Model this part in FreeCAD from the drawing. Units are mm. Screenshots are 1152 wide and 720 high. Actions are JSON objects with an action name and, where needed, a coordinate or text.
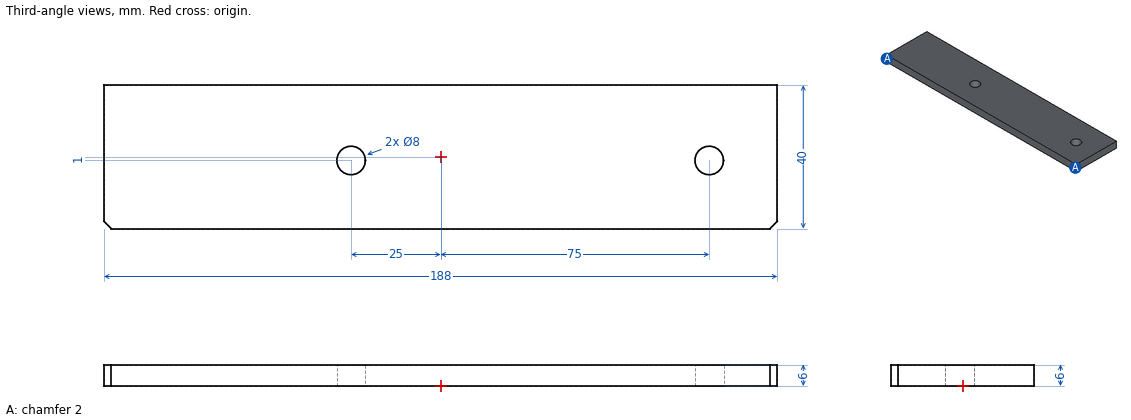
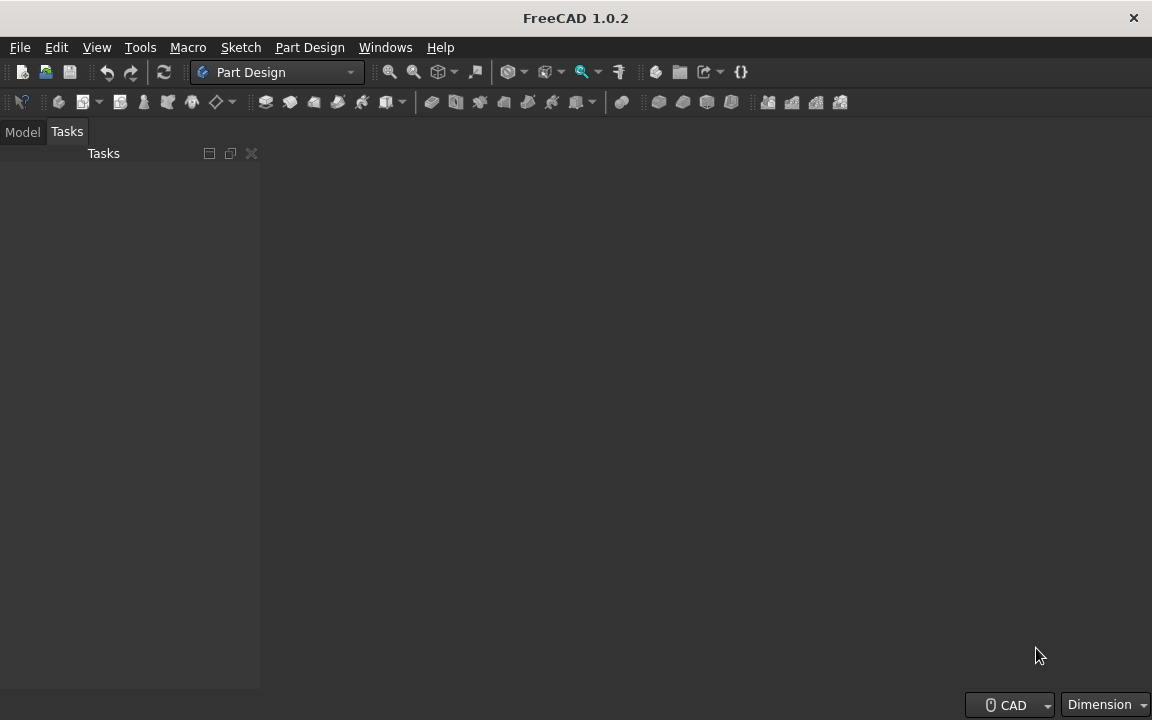
{"action": "key", "text": "ctrl+n"}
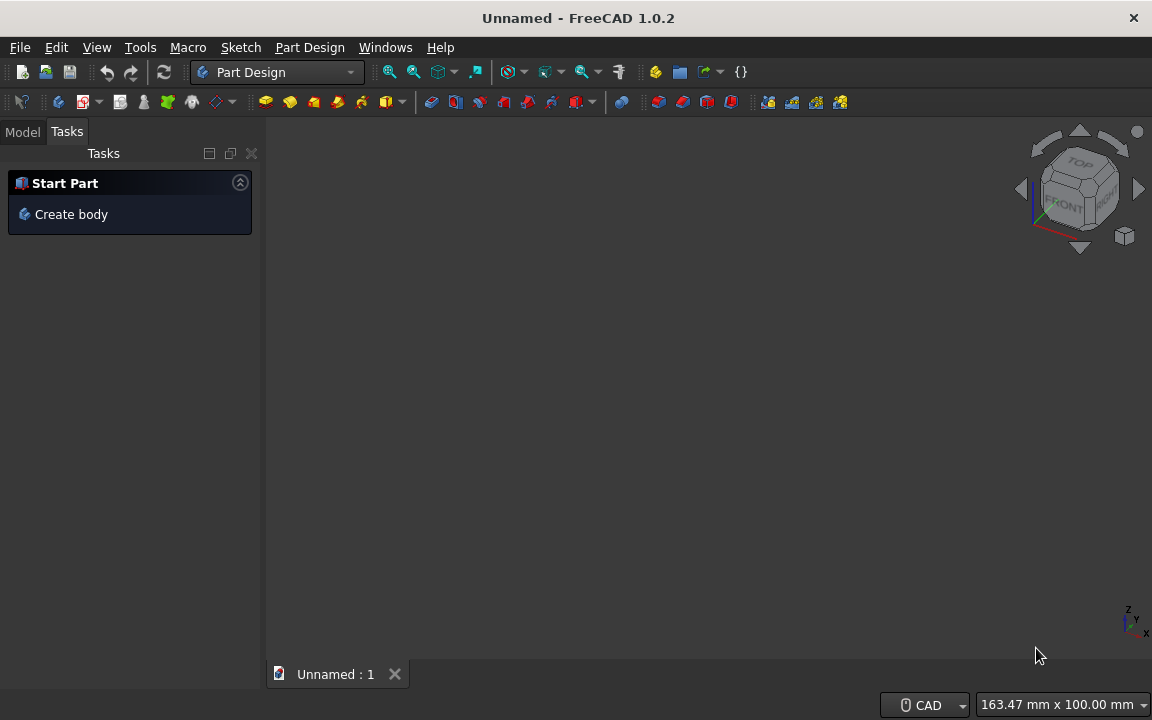
{"action": "left_click", "coordinate": [84, 102]}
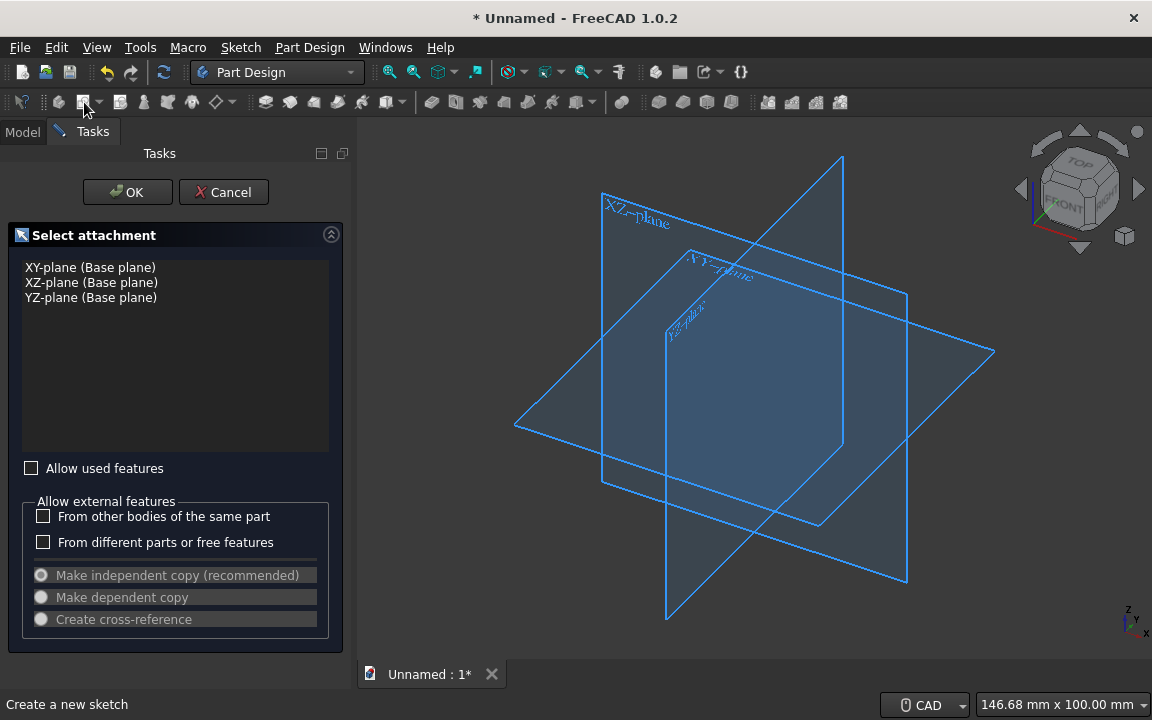
{"action": "left_click", "coordinate": [82, 268]}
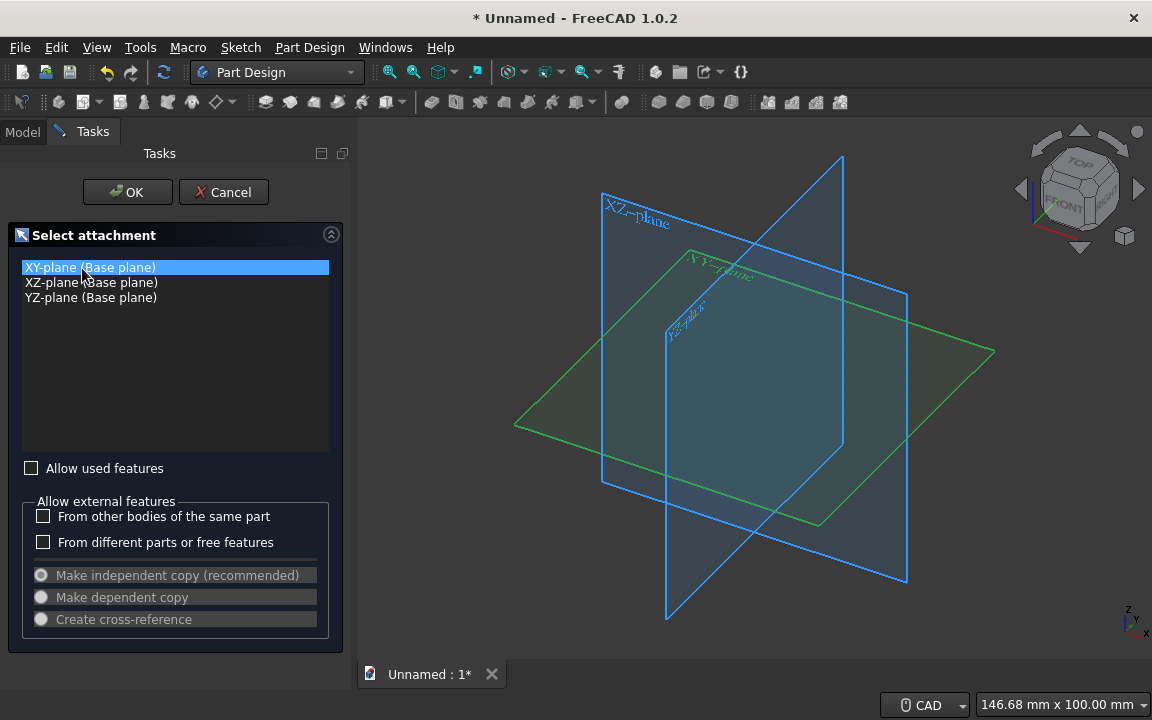
{"action": "left_click", "coordinate": [128, 192]}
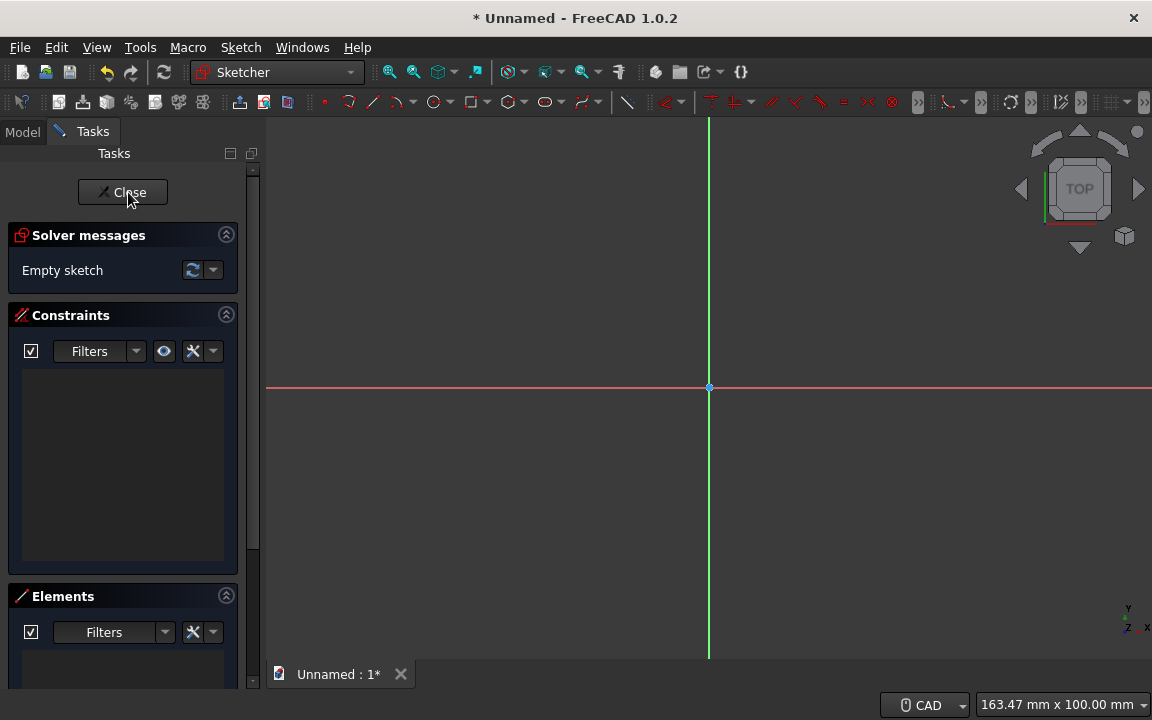
{"action": "scroll", "coordinate": [585, 388], "scroll_direction": "down", "scroll_amount": 4}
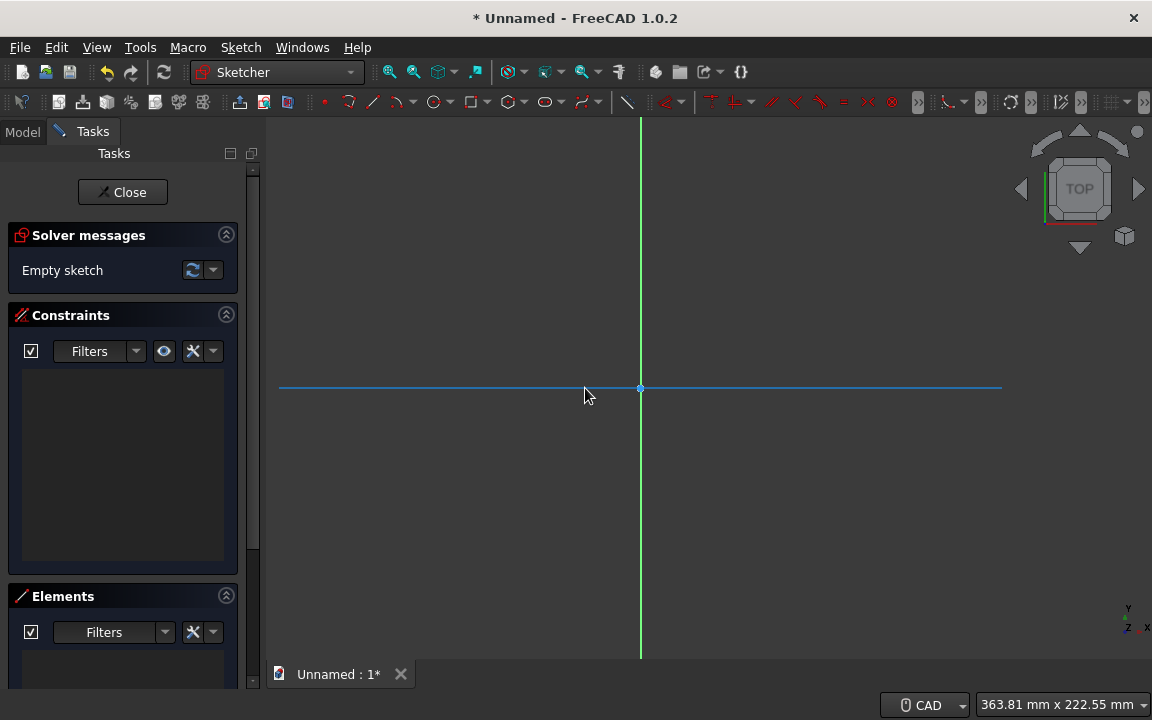
{"action": "left_click", "coordinate": [490, 102]}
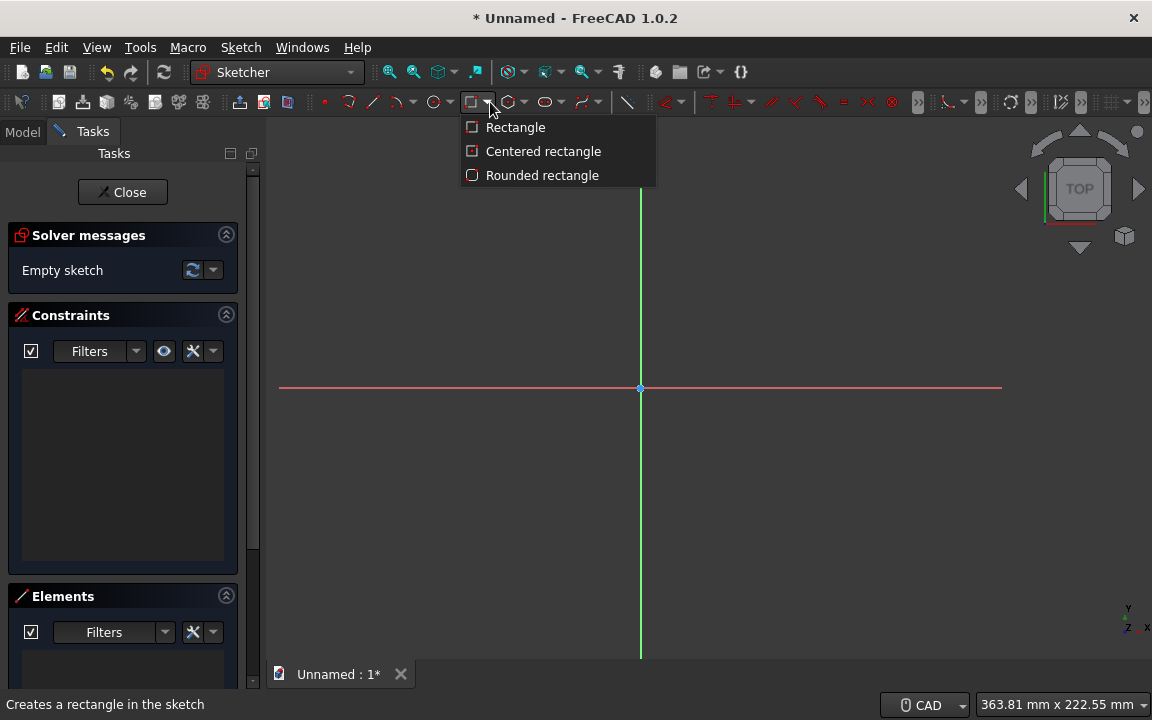
{"action": "left_click", "coordinate": [558, 151]}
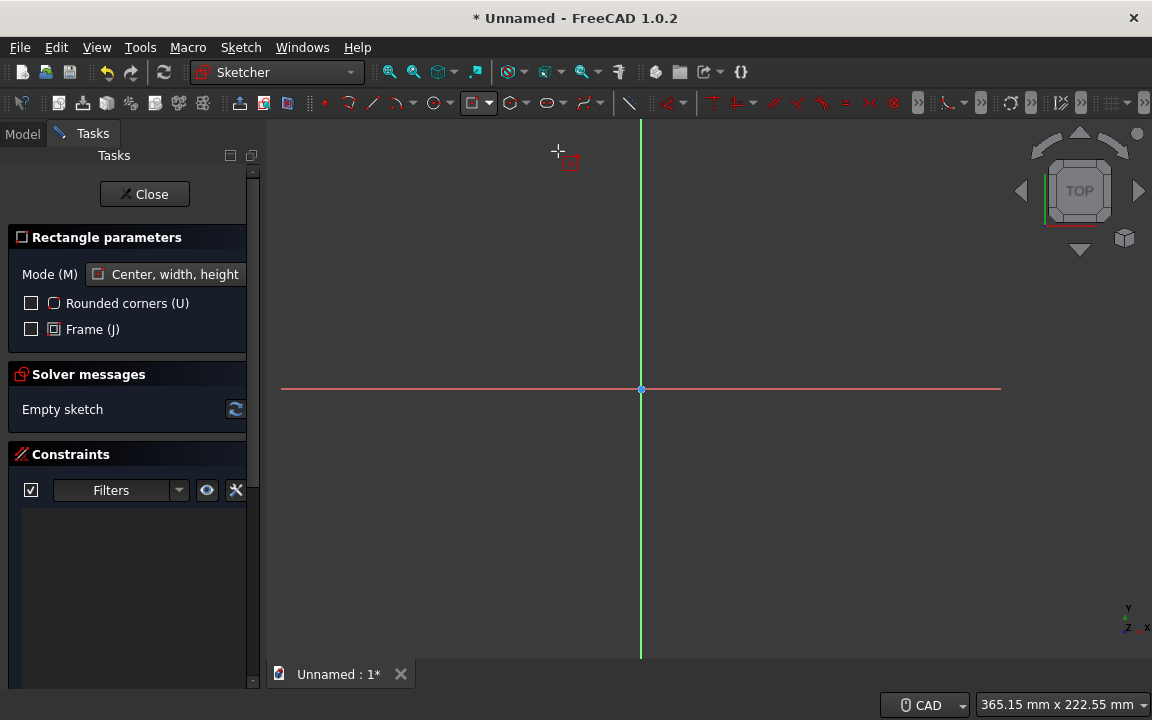
{"action": "left_click", "coordinate": [641, 389]}
{"action": "mouse_move", "coordinate": [869, 341]}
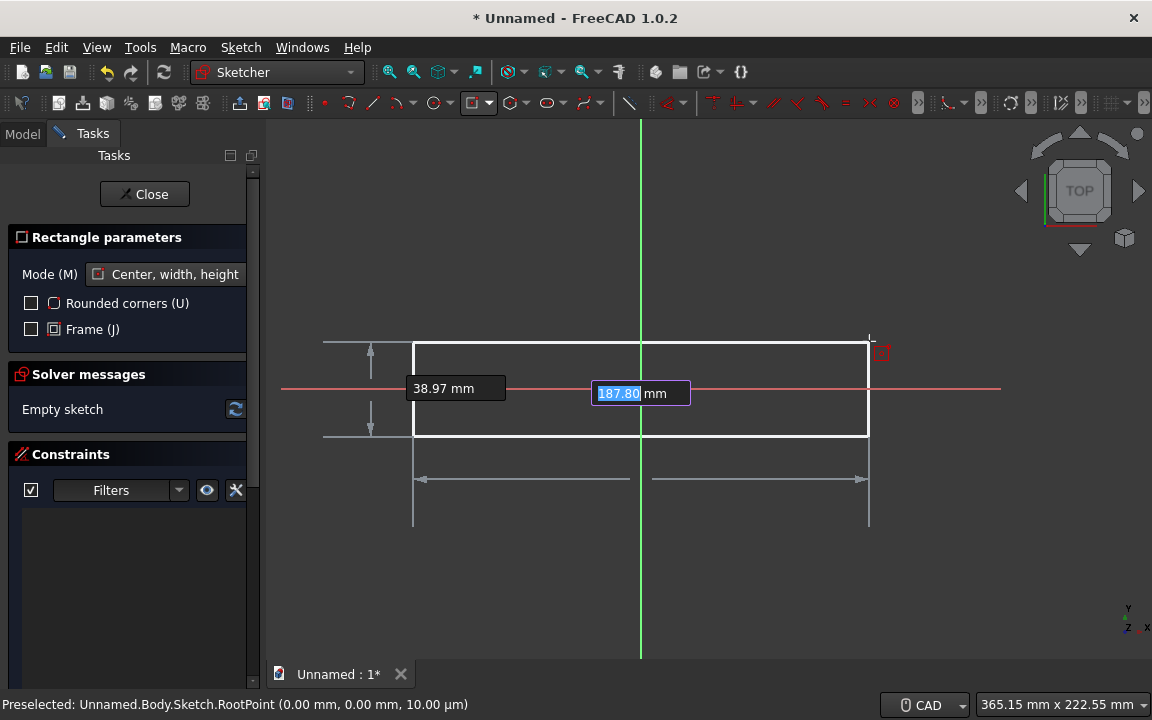
{"action": "type", "text": "188"}
{"action": "key", "text": "Tab"}
{"action": "type", "text": "40"}
{"action": "key", "text": "Return"}
{"action": "key", "text": "Escape"}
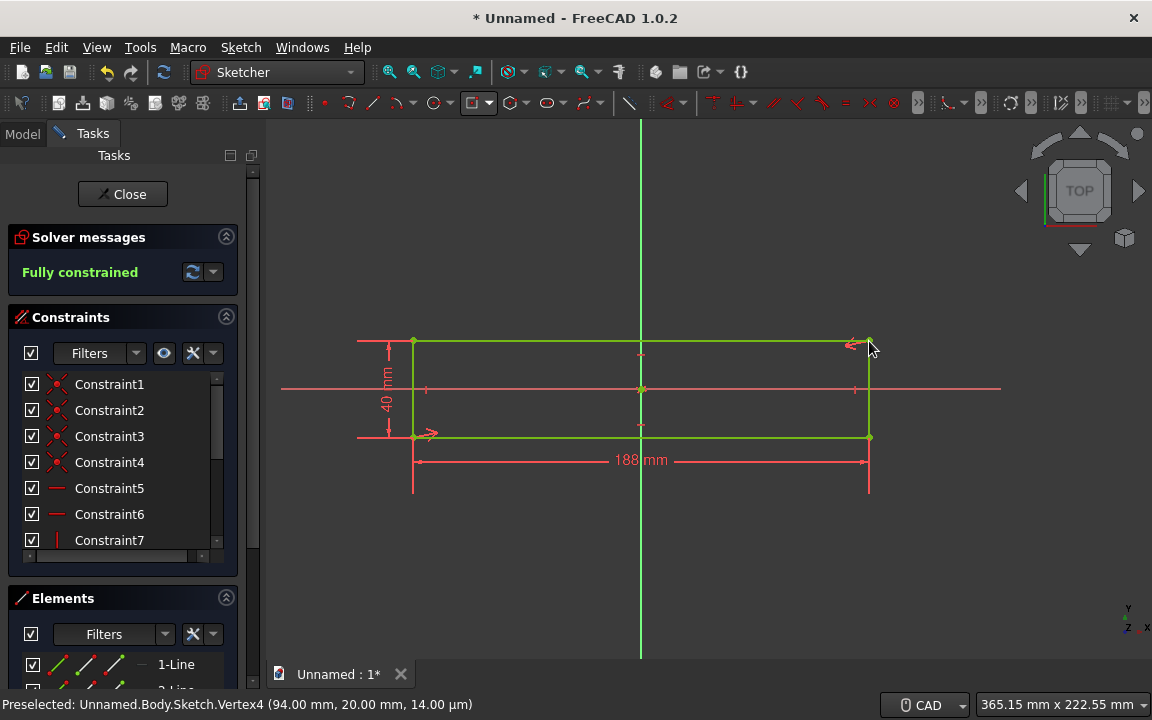
{"action": "left_click", "coordinate": [123, 194]}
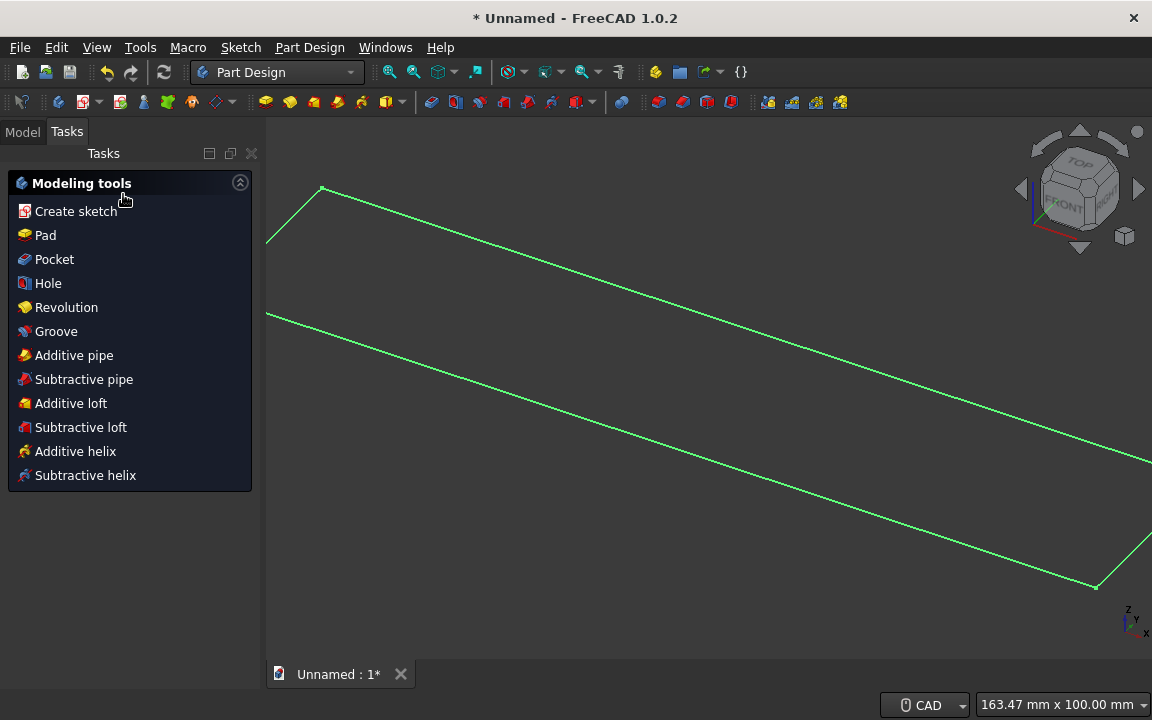
{"action": "left_click", "coordinate": [266, 102]}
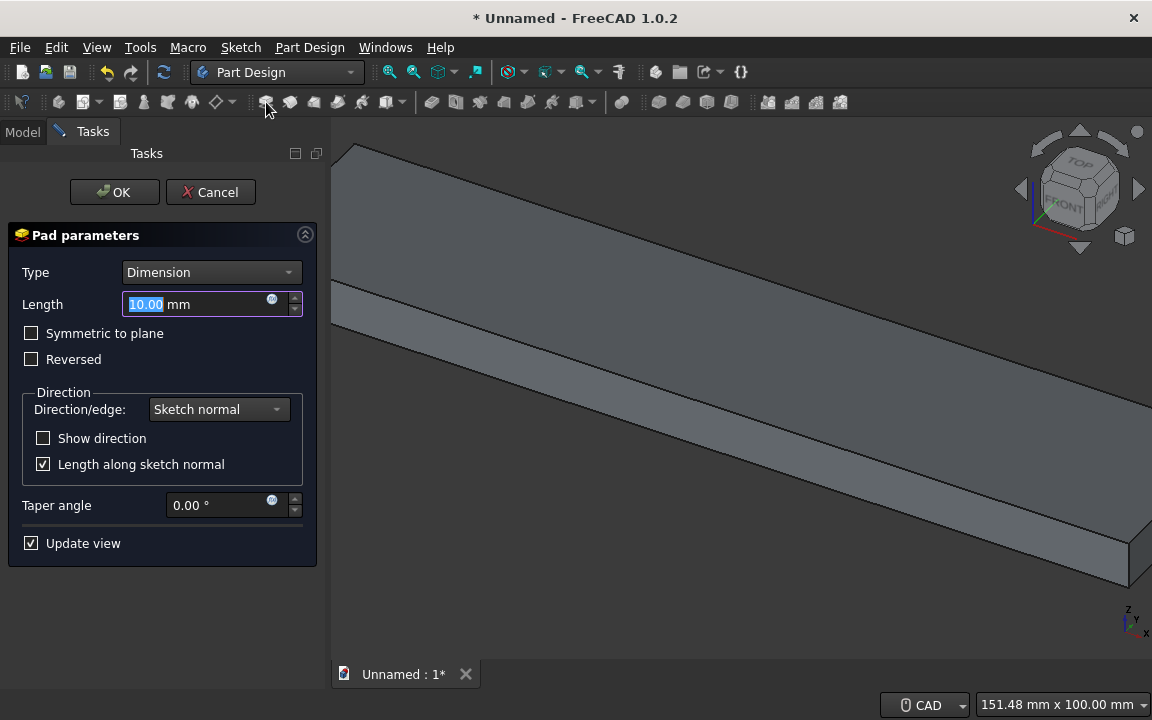
{"action": "type", "text": "6"}
{"action": "key", "text": "Tab"}